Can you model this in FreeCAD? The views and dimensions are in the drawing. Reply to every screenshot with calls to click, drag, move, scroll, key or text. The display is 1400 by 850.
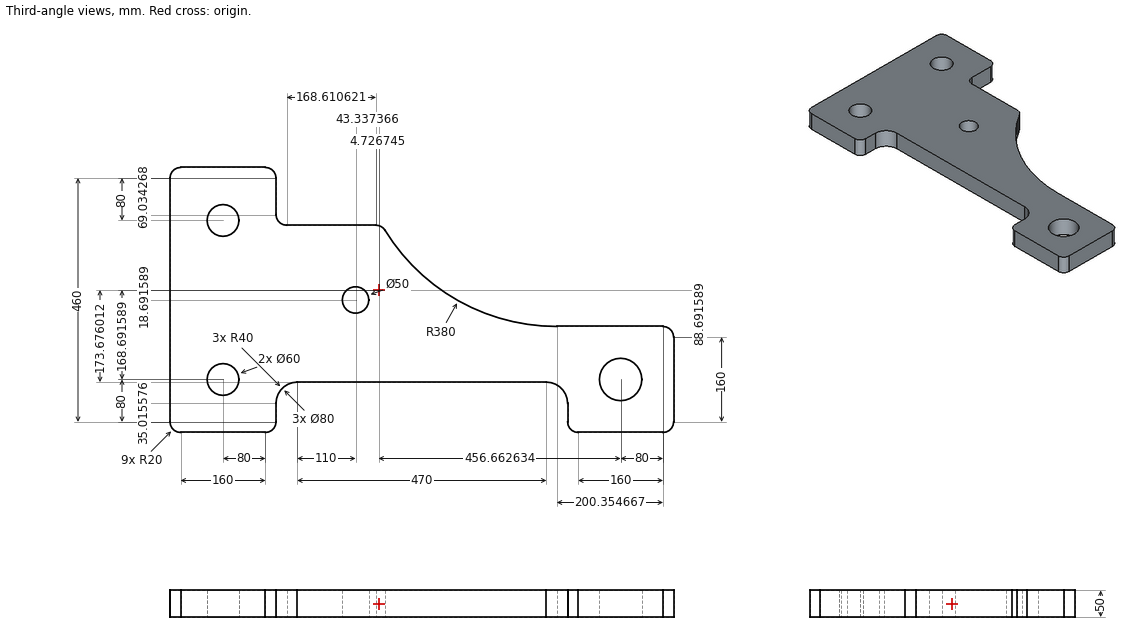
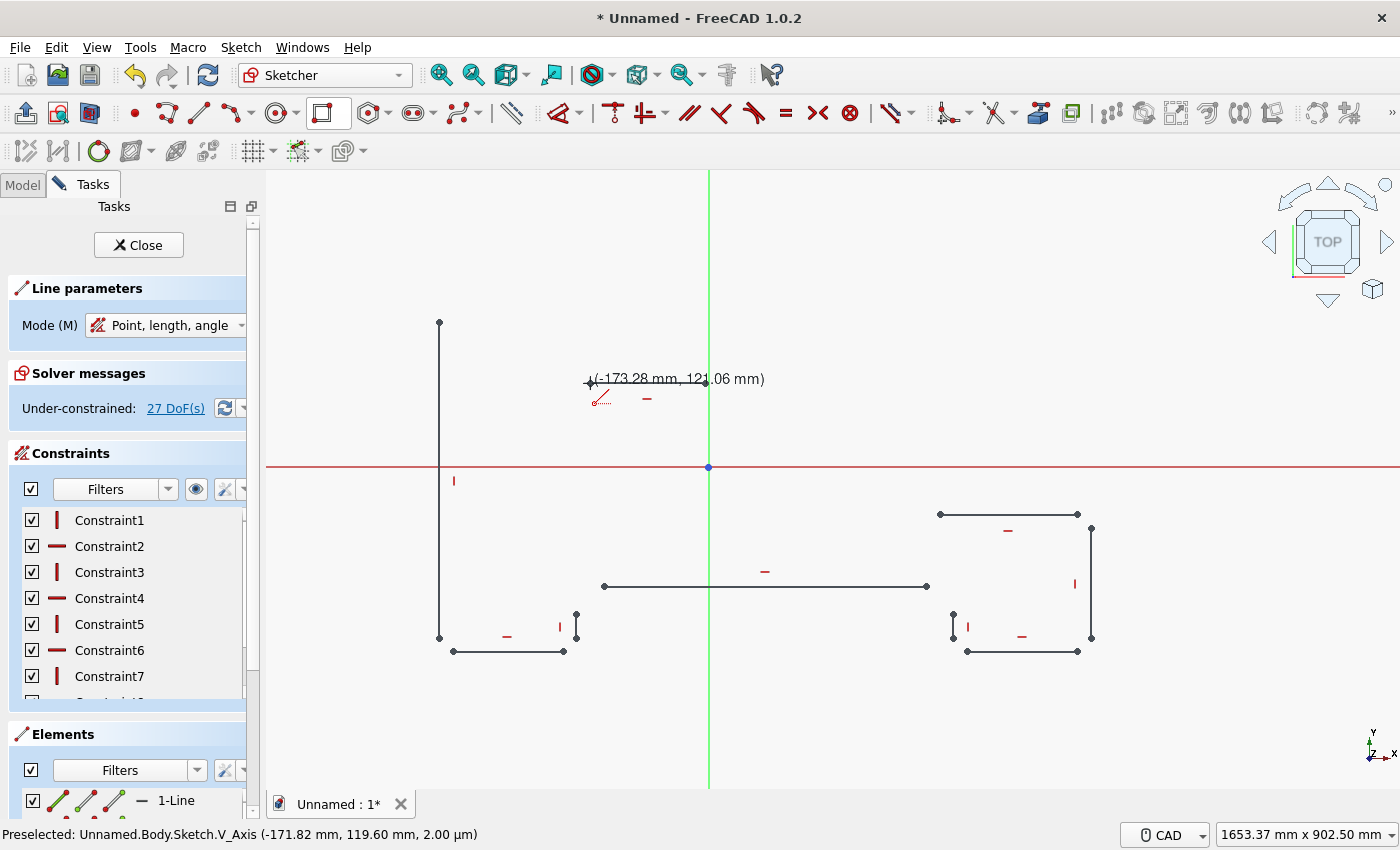
click(576, 369)
click(576, 322)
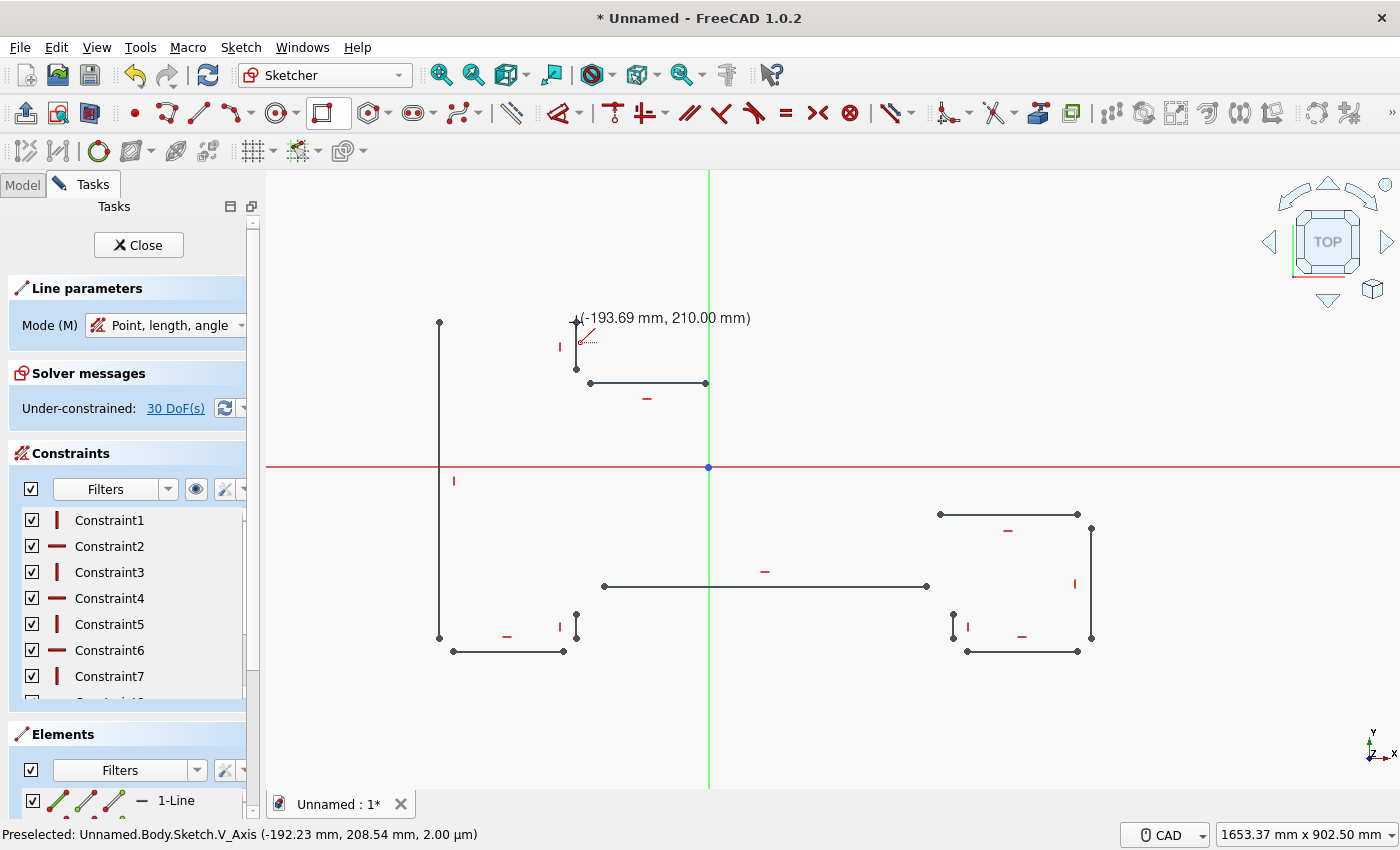
click(563, 308)
click(453, 308)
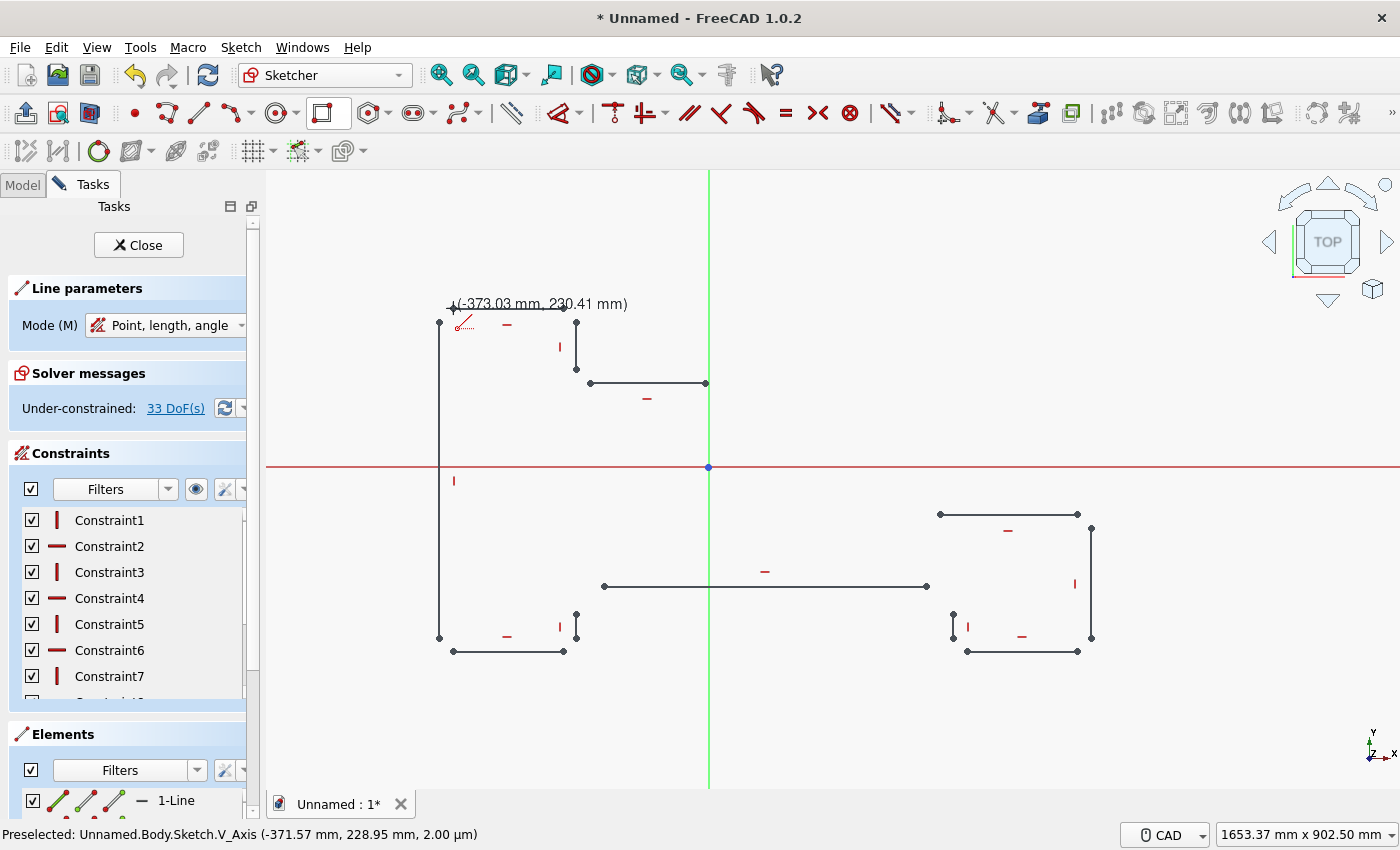
click(232, 114)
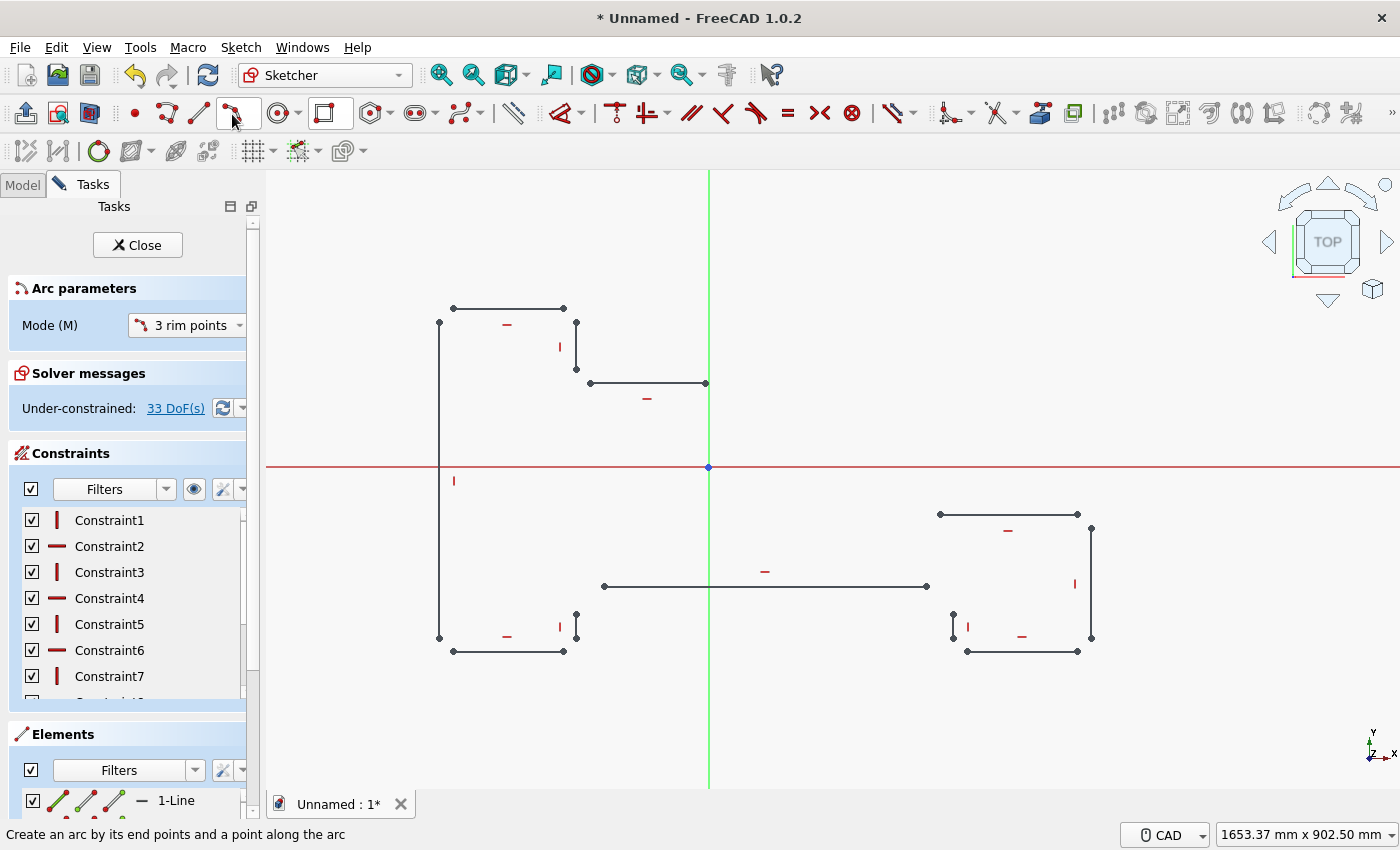
click(439, 639)
click(453, 652)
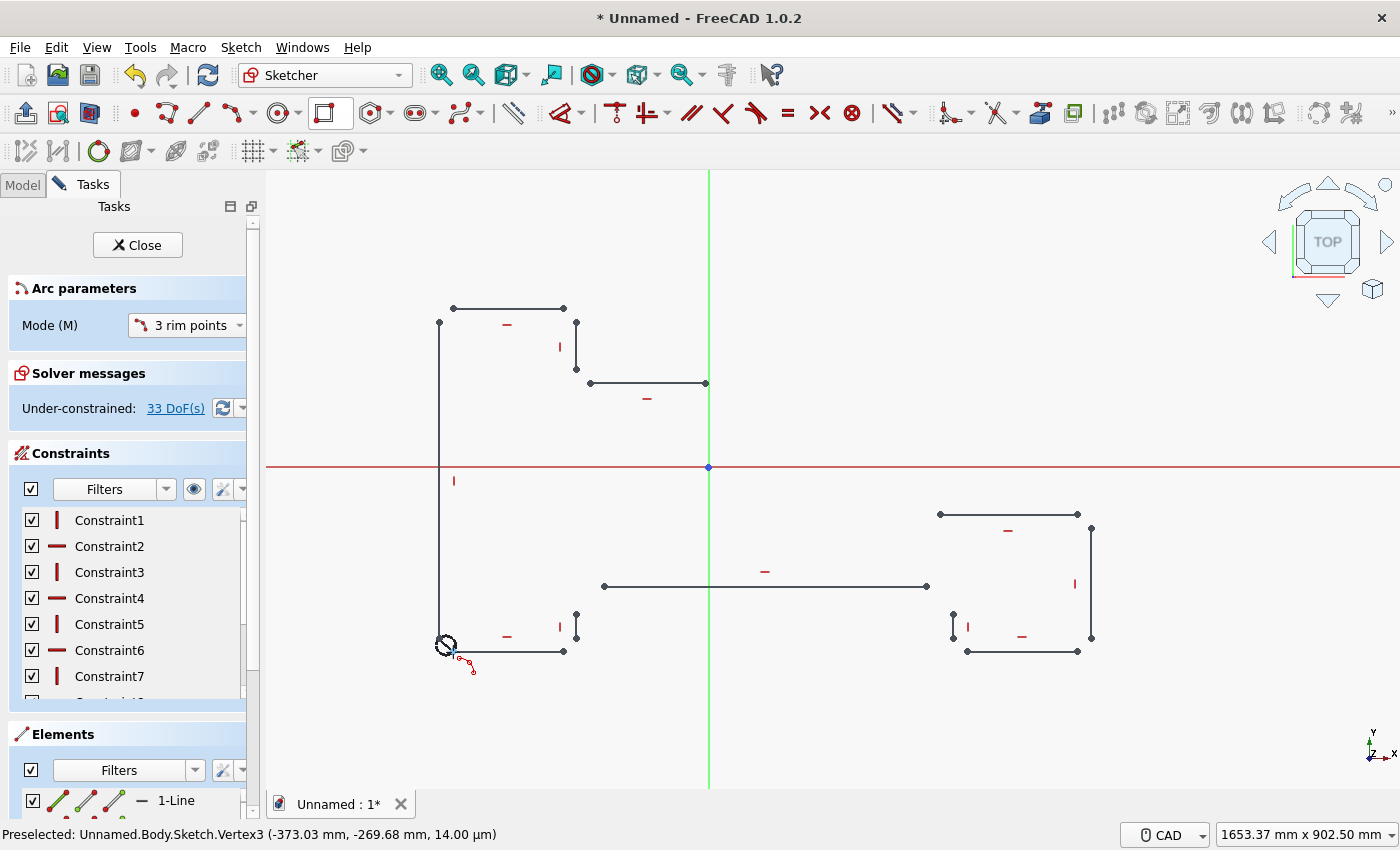
scroll(443, 647, up, 7)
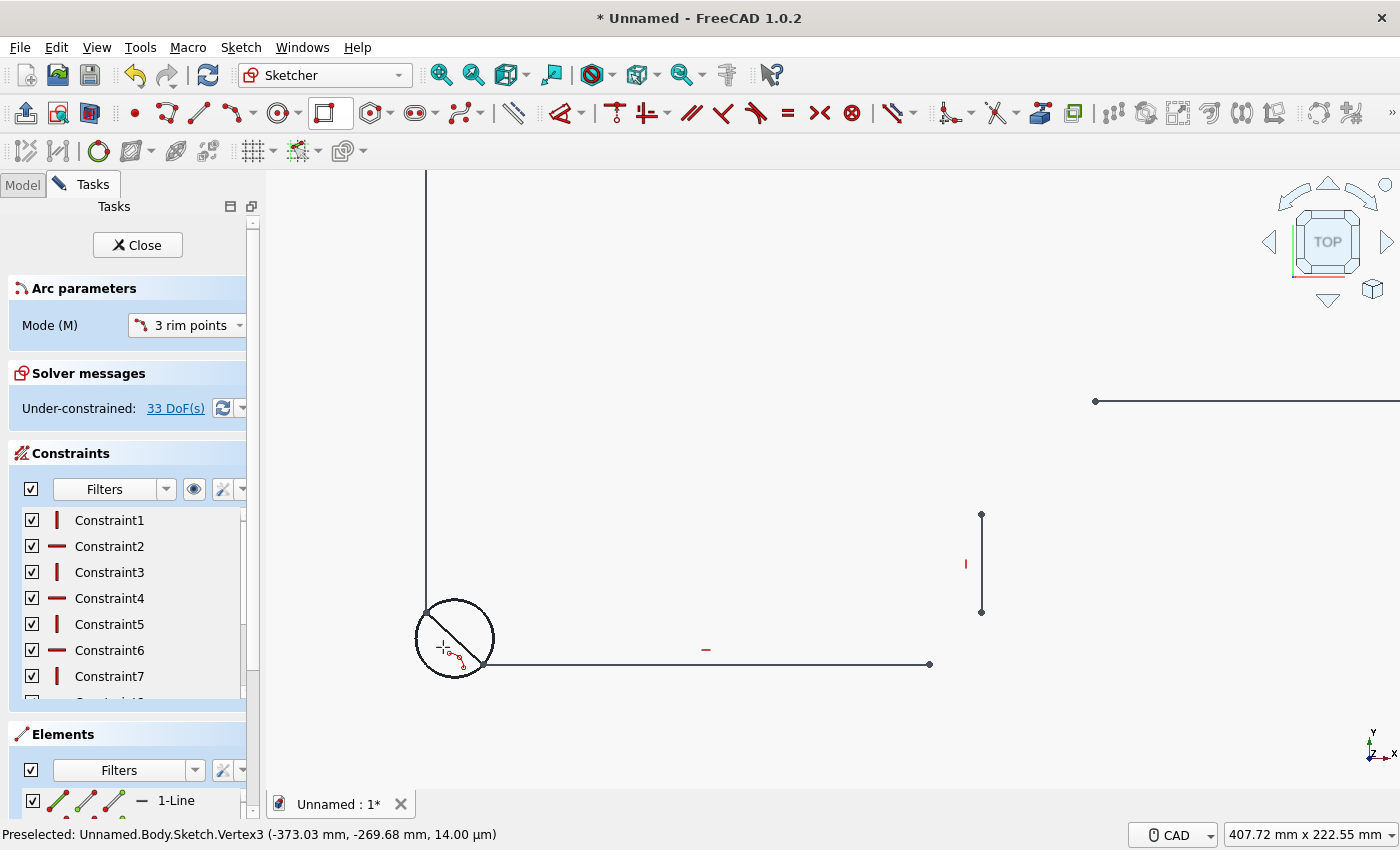
click(443, 646)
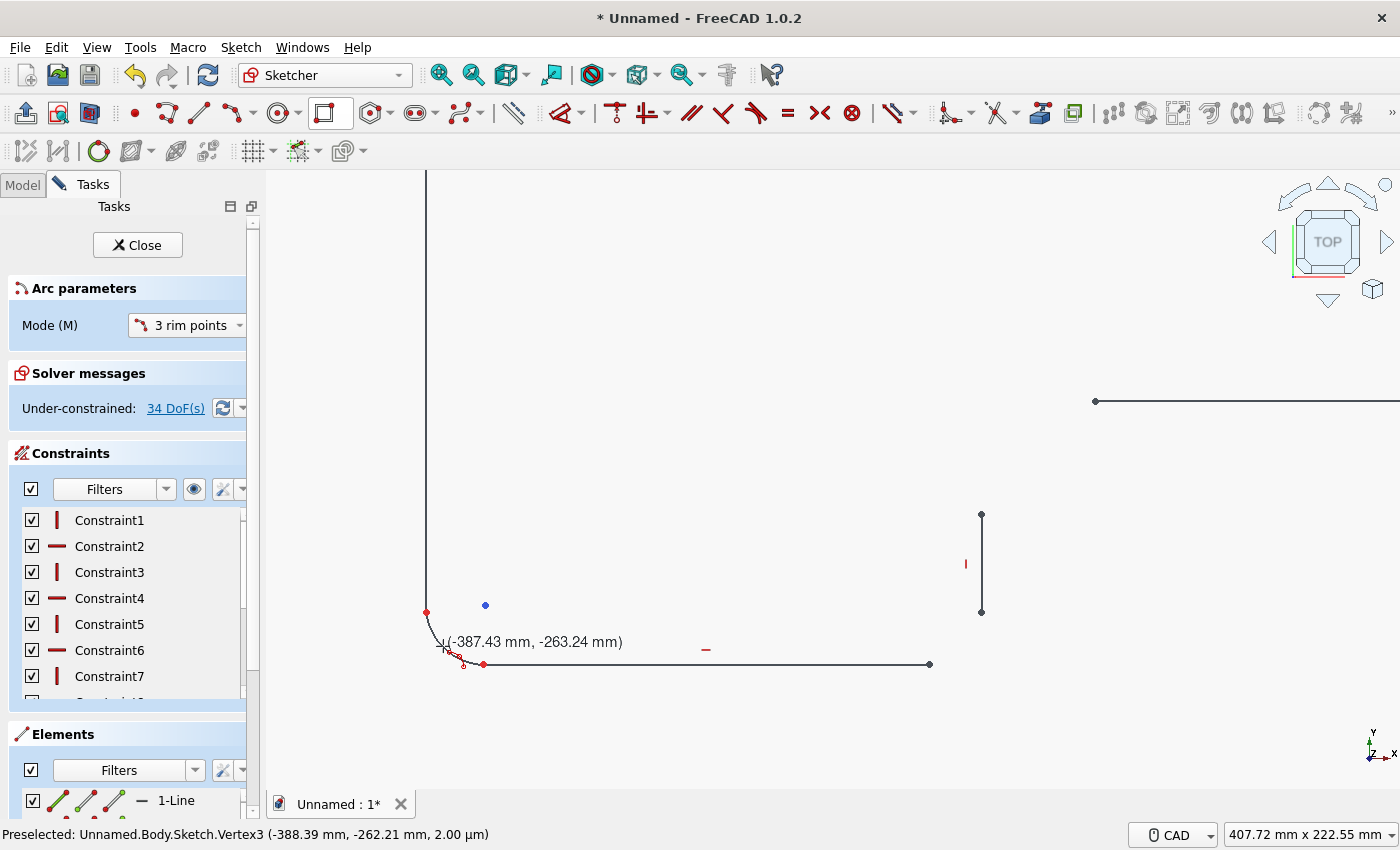
scroll(443, 647, down, 7)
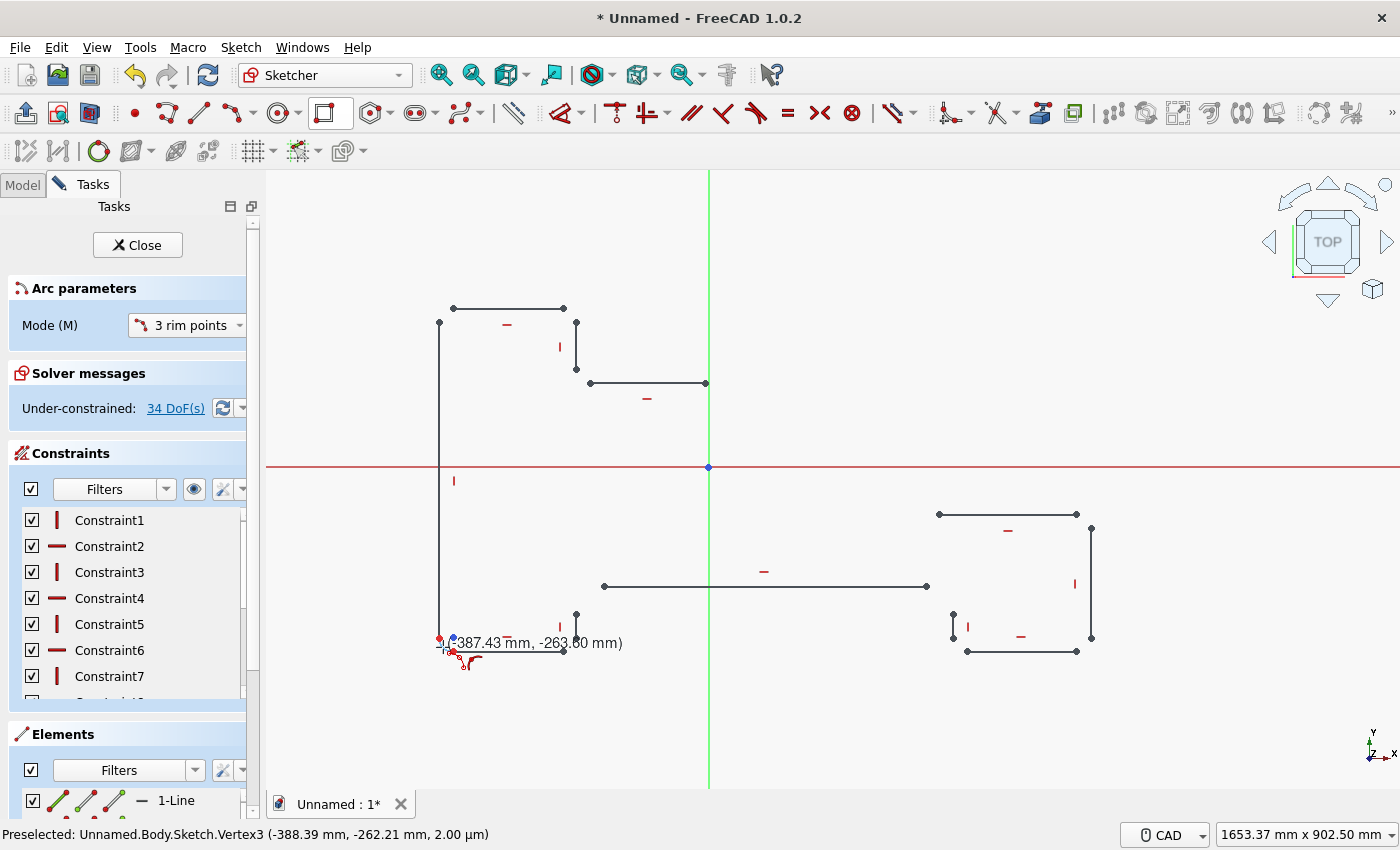
click(563, 652)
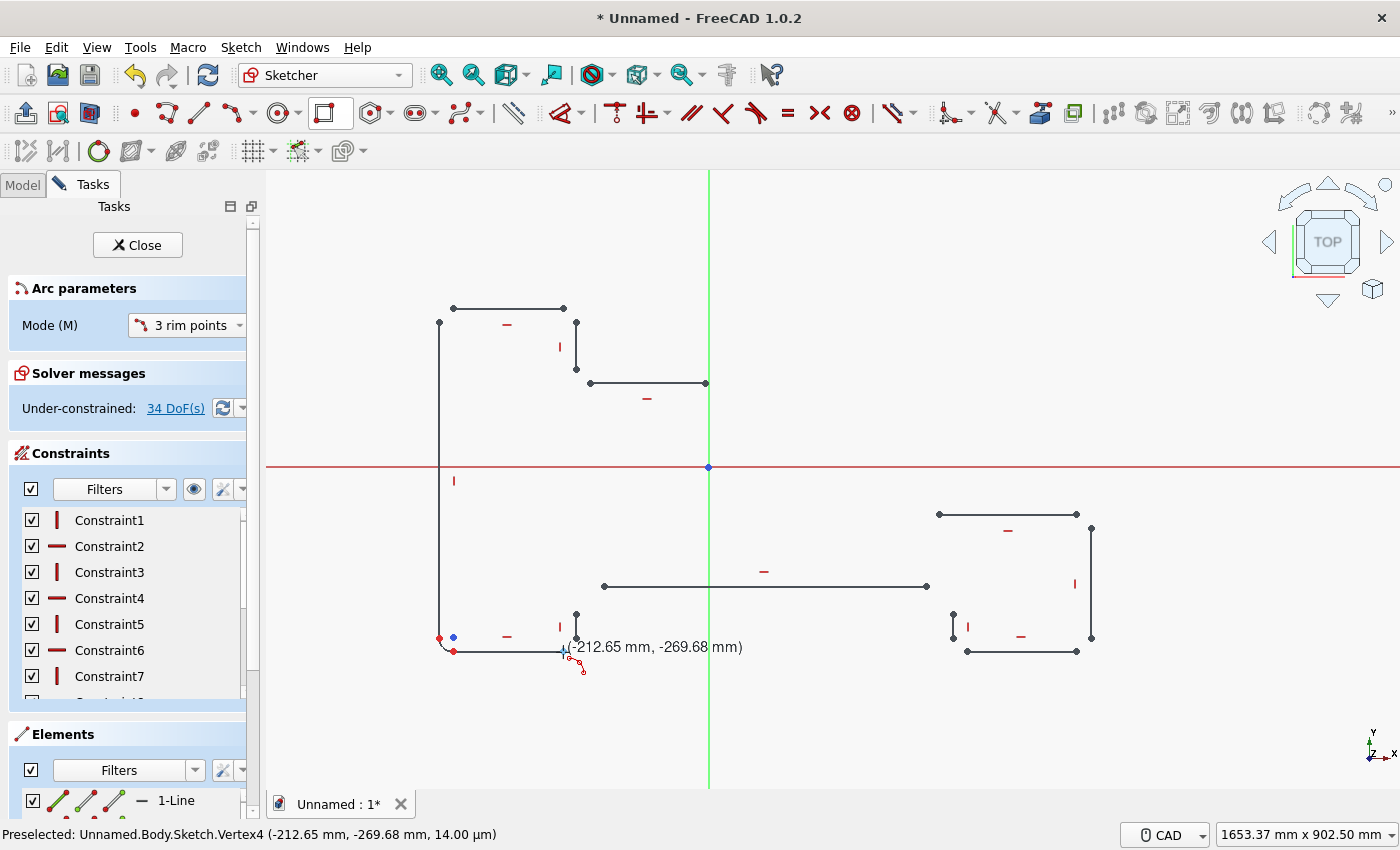
scroll(576, 638, up, 2)